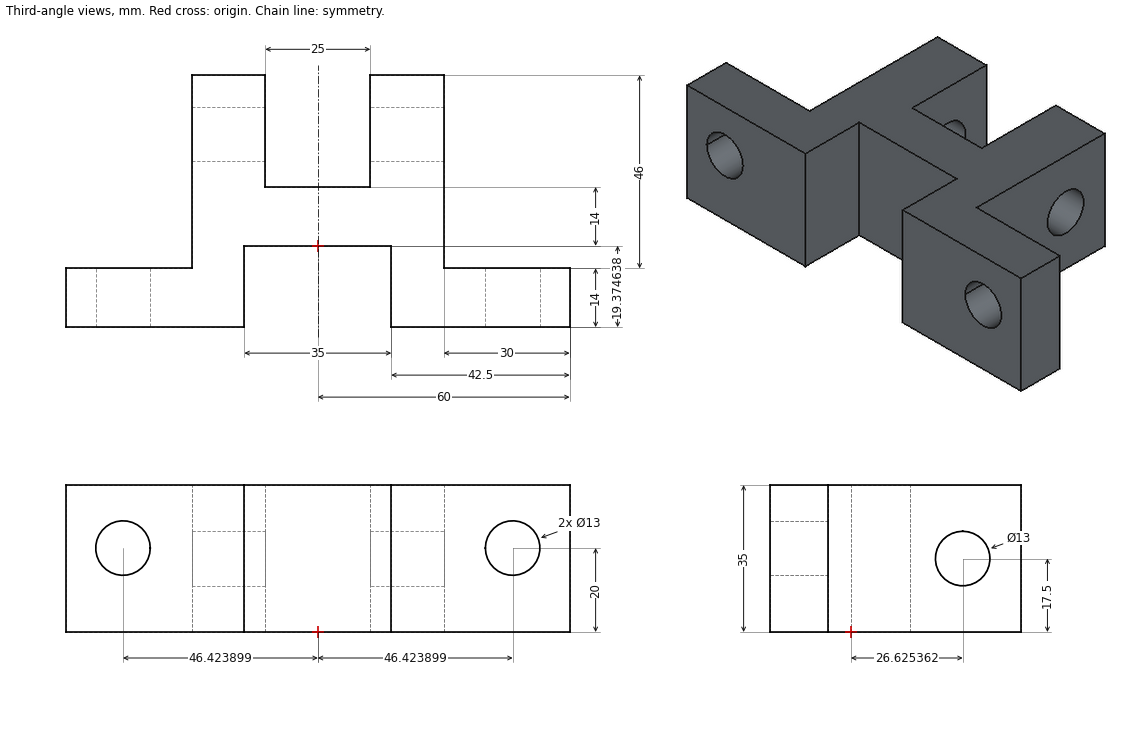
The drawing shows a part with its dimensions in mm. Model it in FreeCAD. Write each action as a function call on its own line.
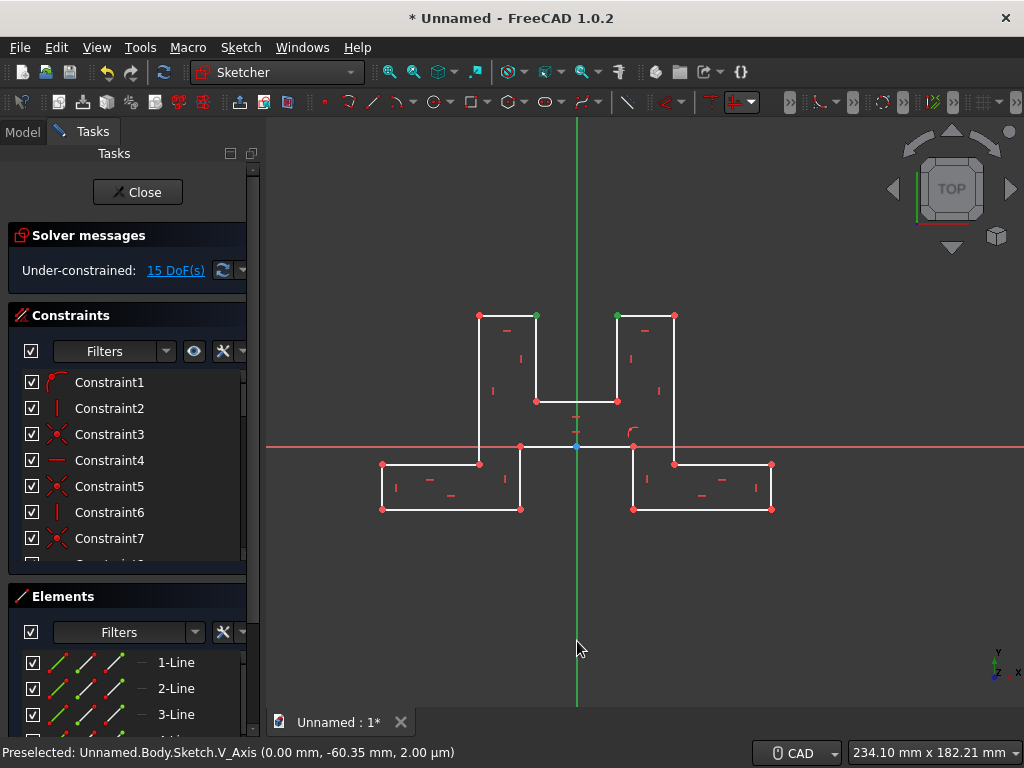
key(s)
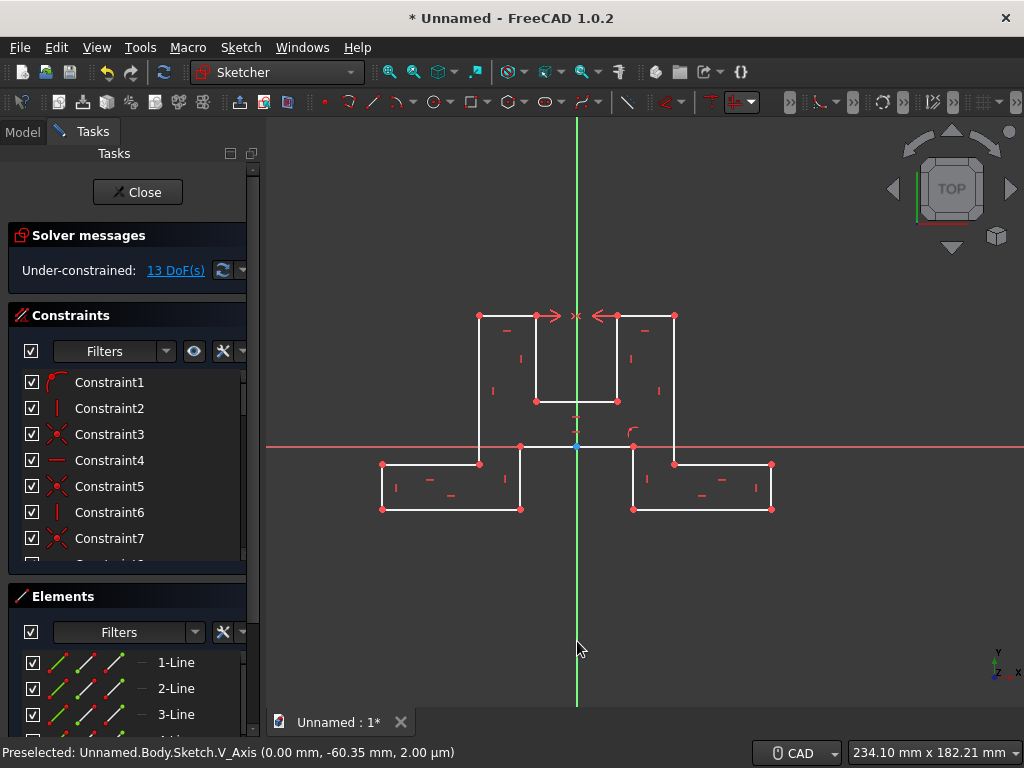
click(674, 465)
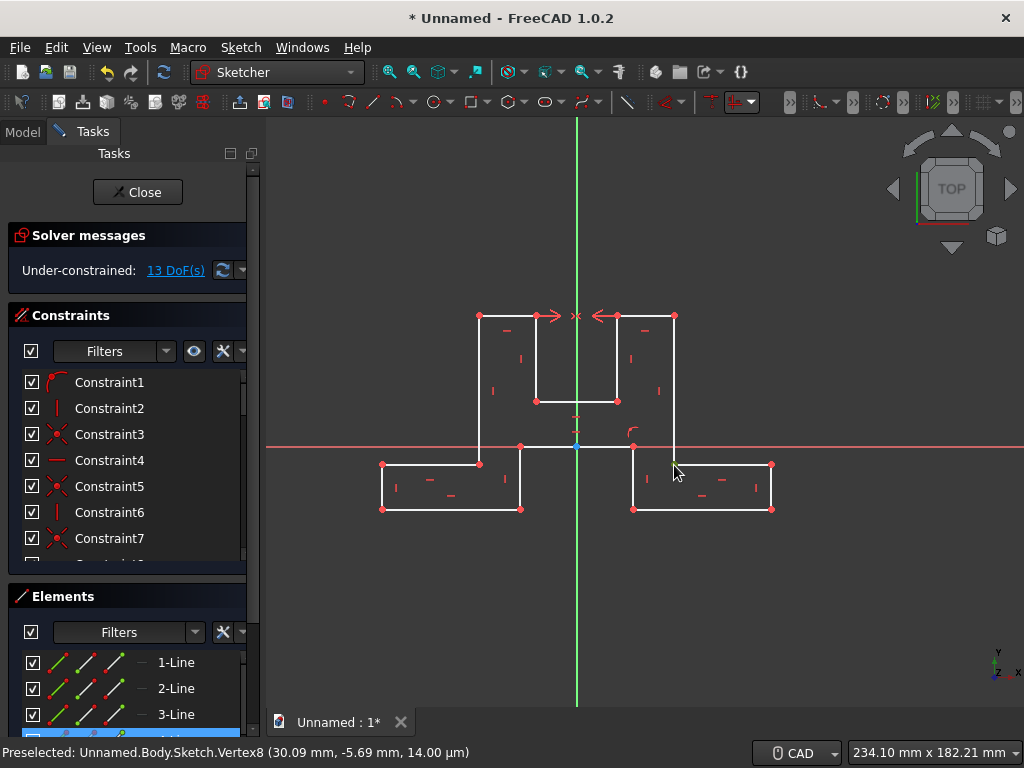
click(479, 465)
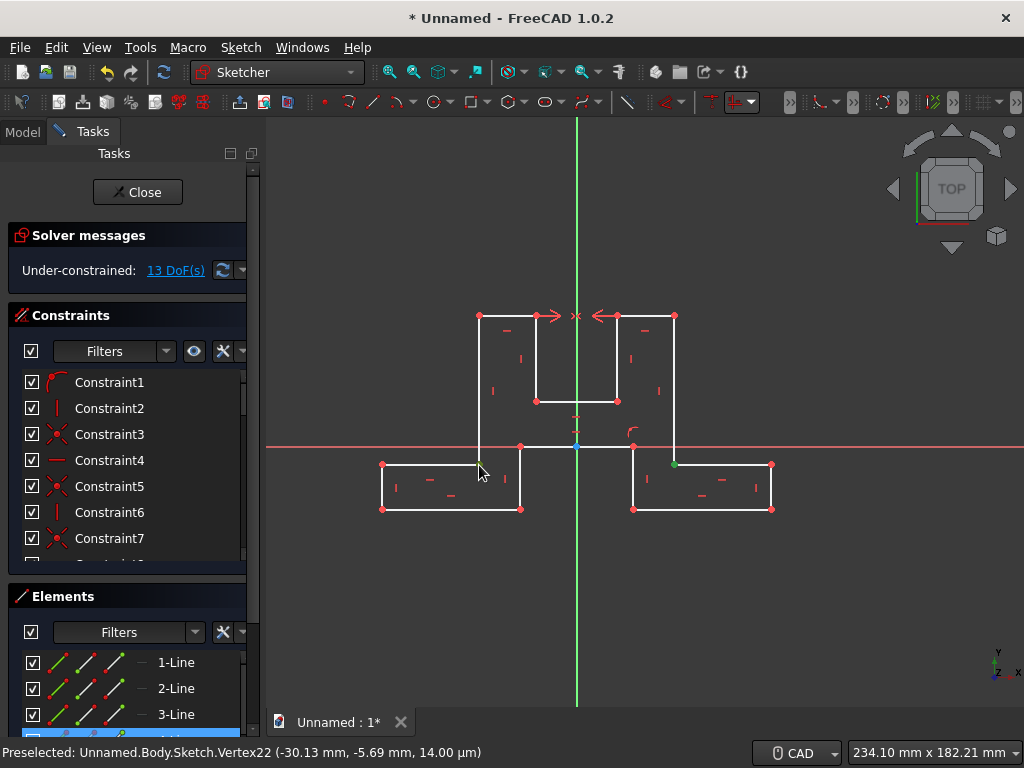
click(577, 641)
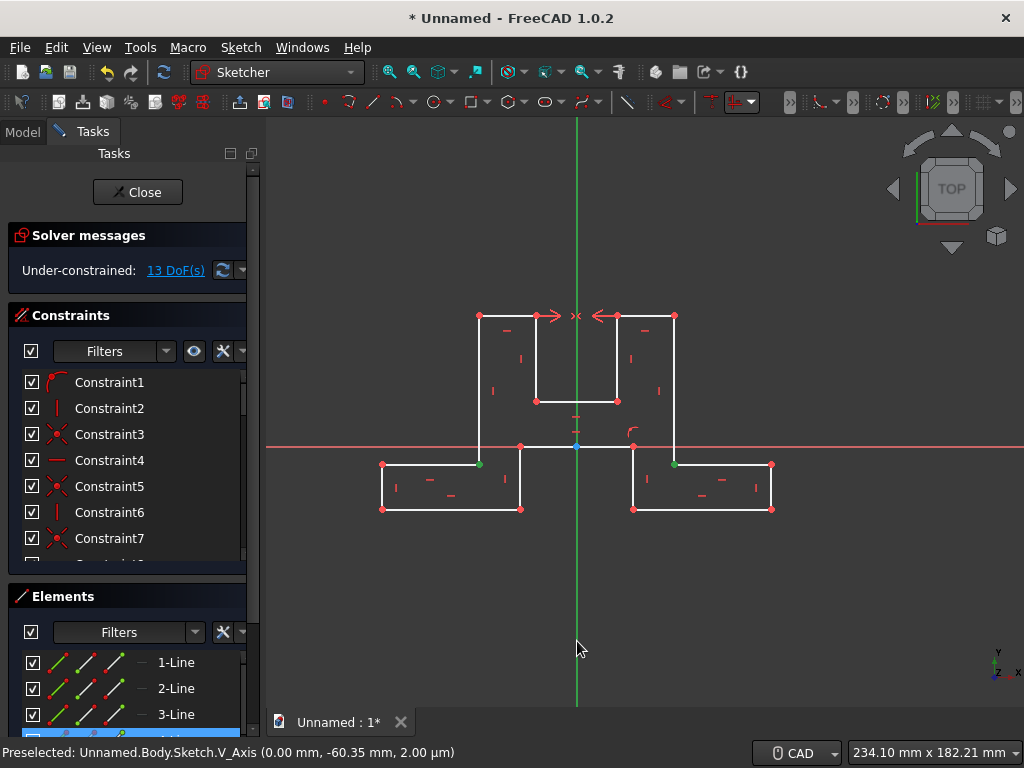
key(s)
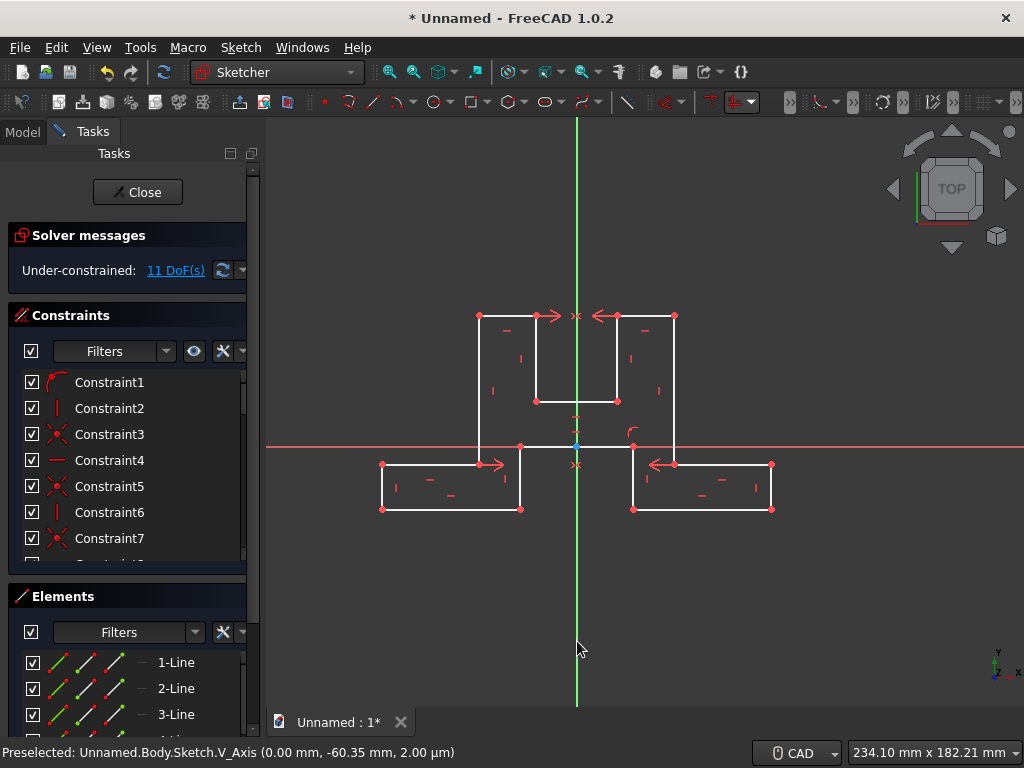
click(771, 510)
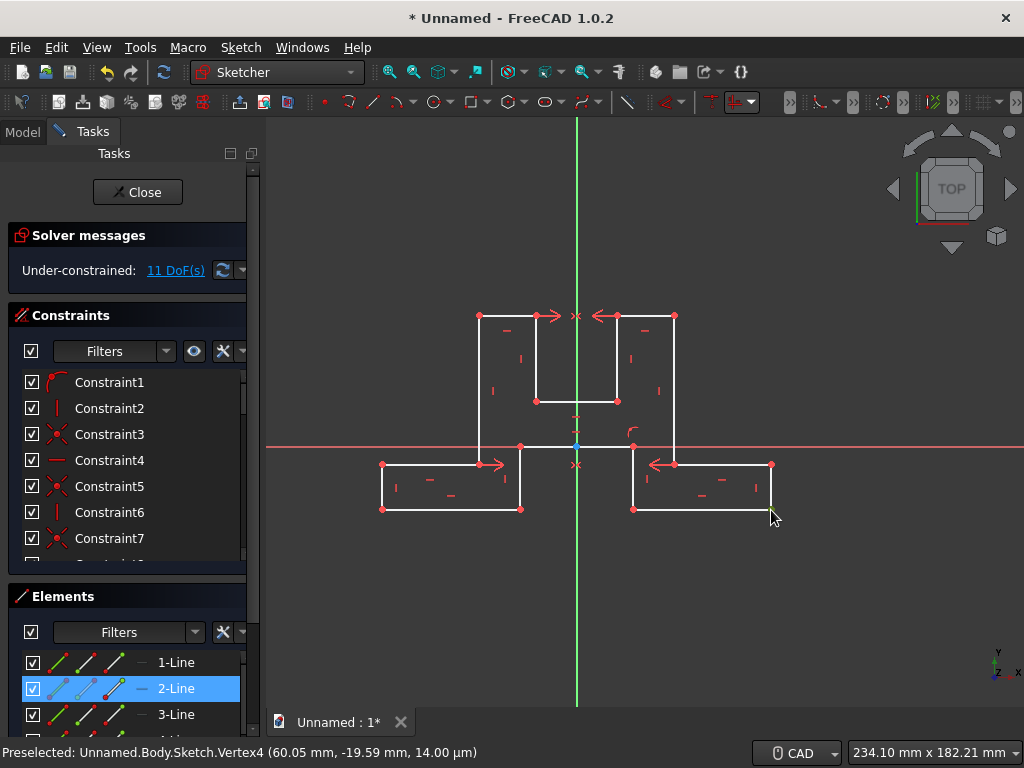
click(382, 510)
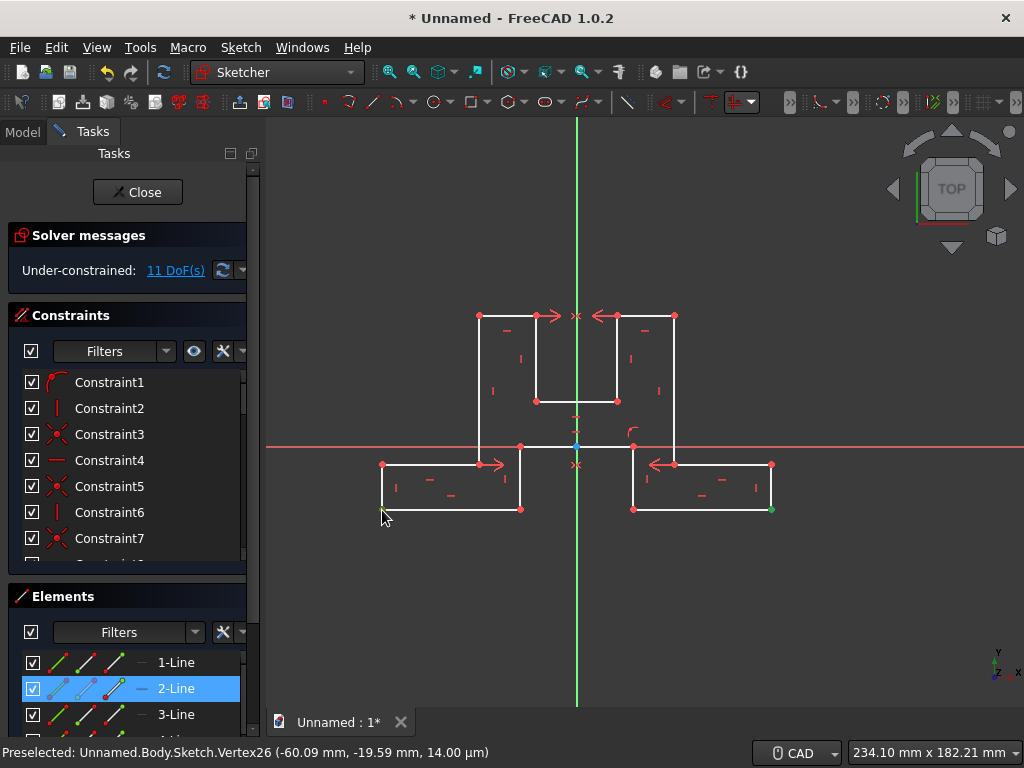
click(577, 641)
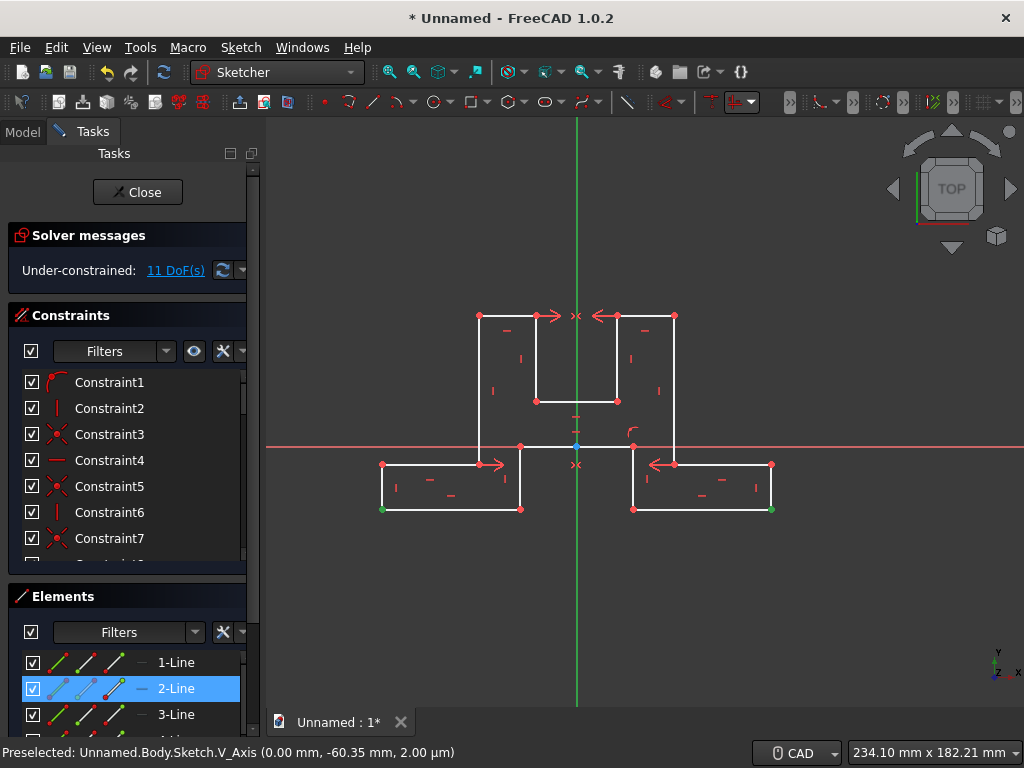
key(s)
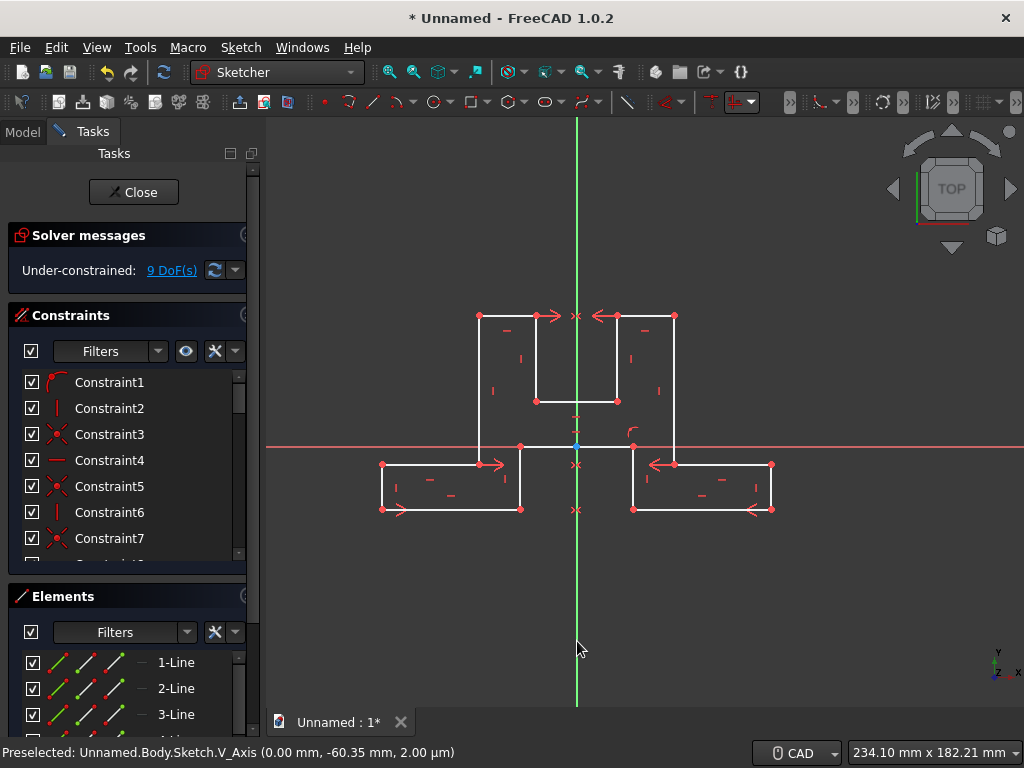
click(666, 102)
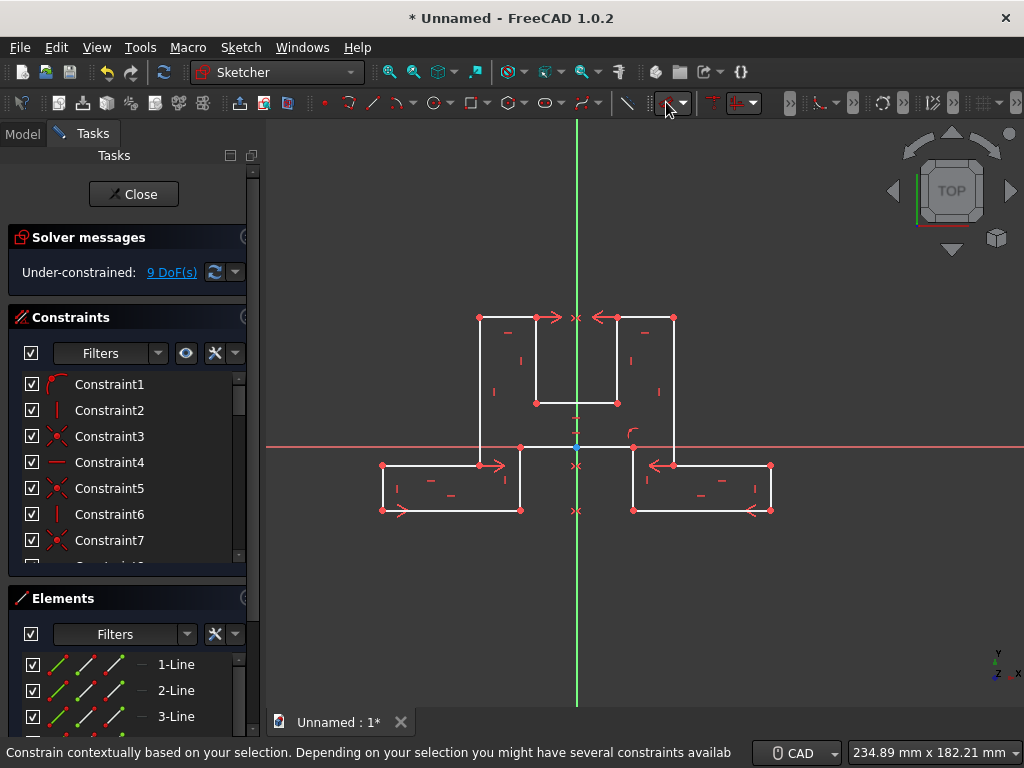
click(771, 497)
click(805, 488)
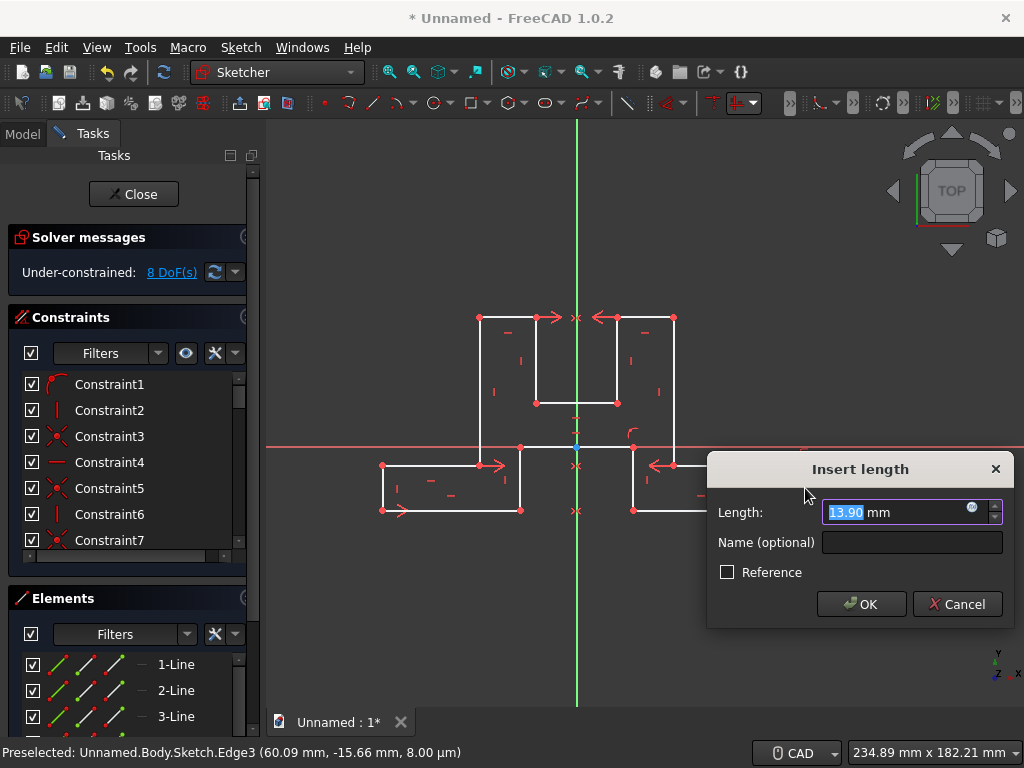
text(14)
key(Return)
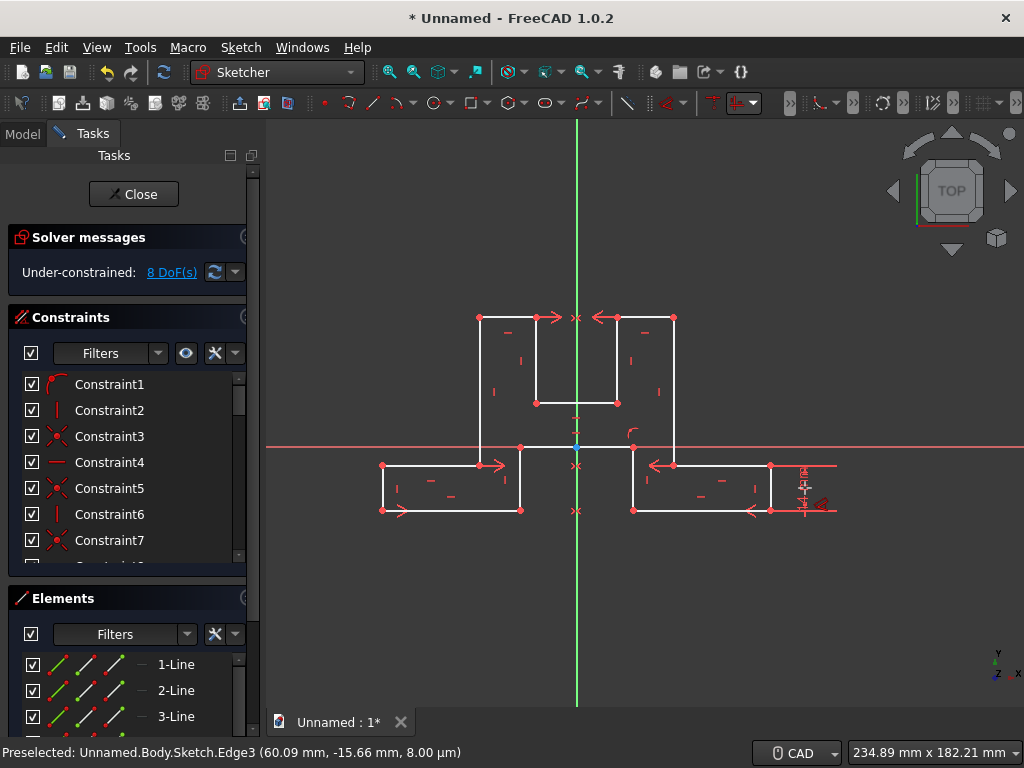
click(742, 466)
click(722, 432)